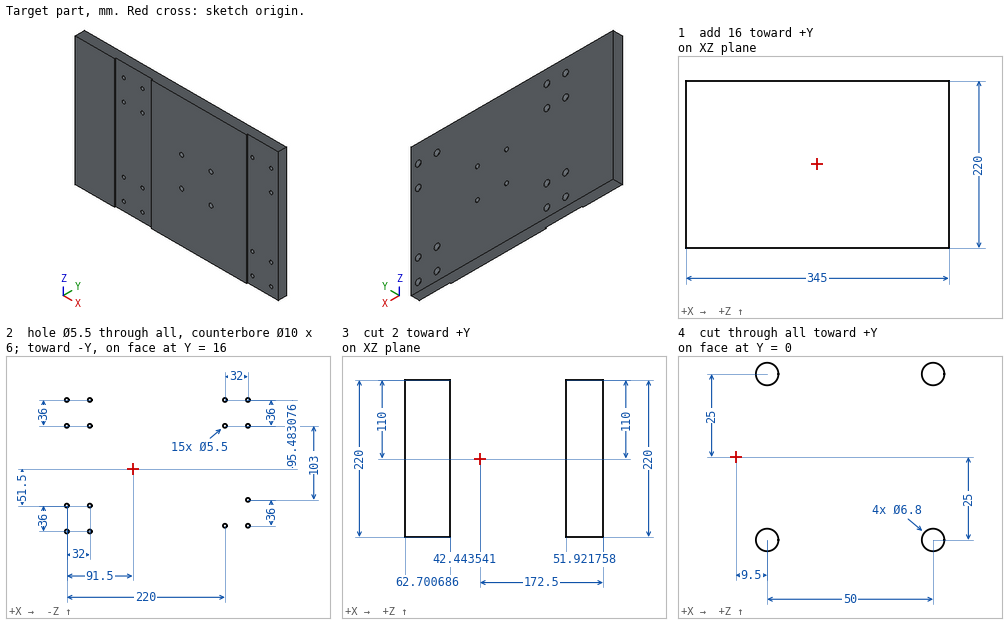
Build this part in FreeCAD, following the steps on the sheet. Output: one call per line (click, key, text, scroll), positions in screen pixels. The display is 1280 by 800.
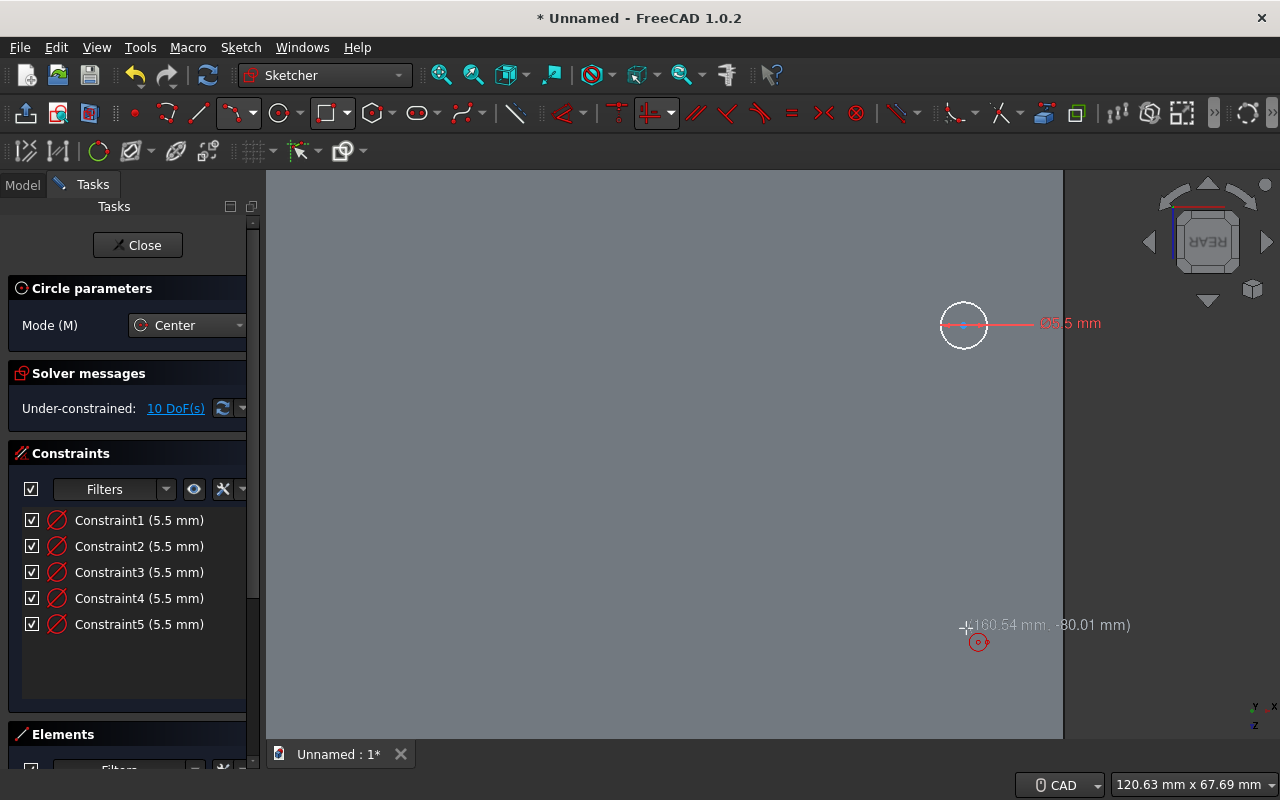
scroll(966, 628, down, 7)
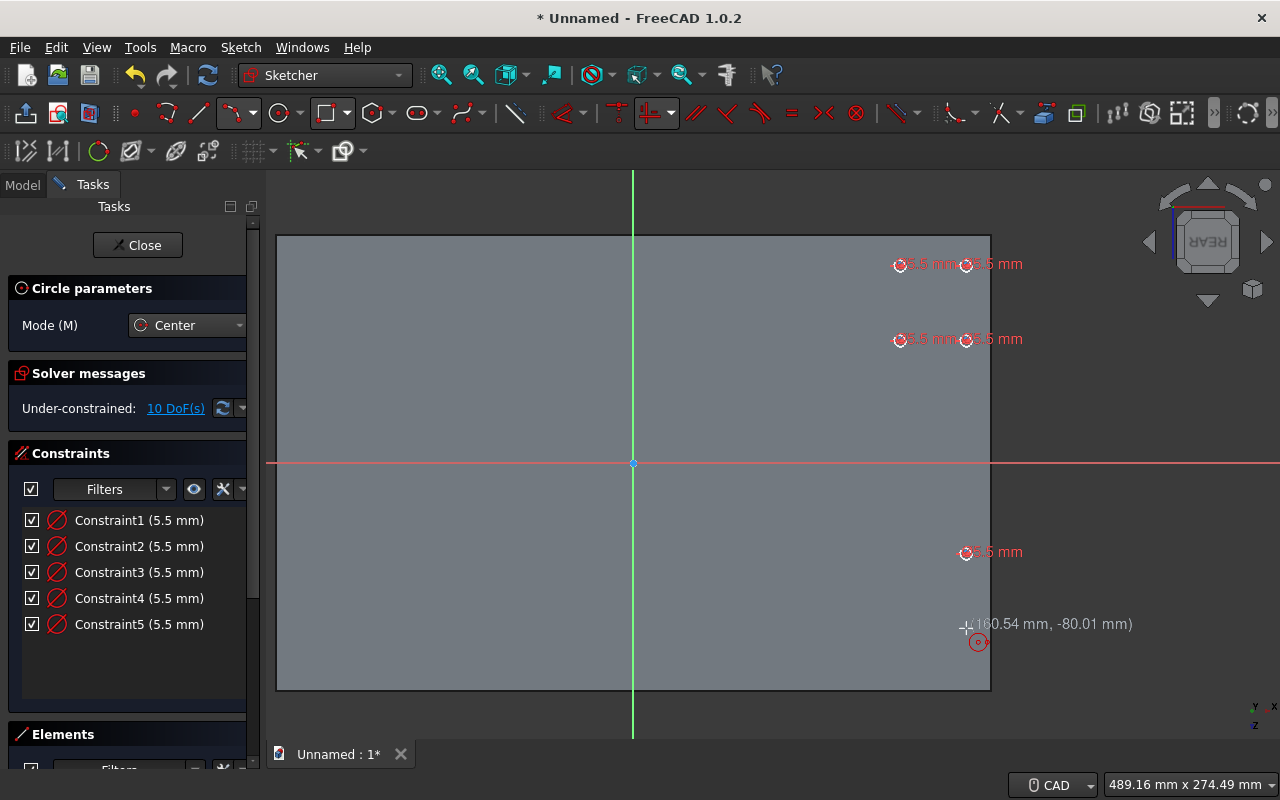
click(966, 628)
move(970, 624)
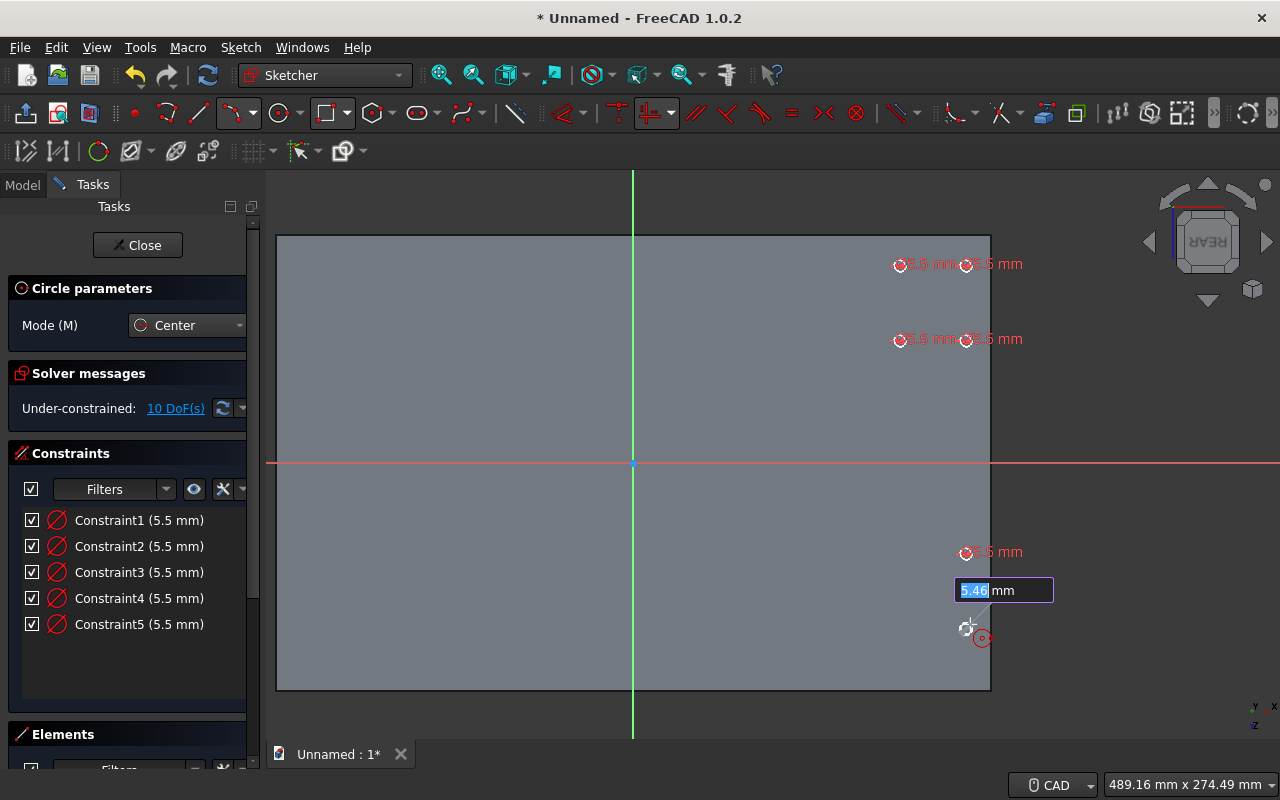
text(5.5)
key(Return)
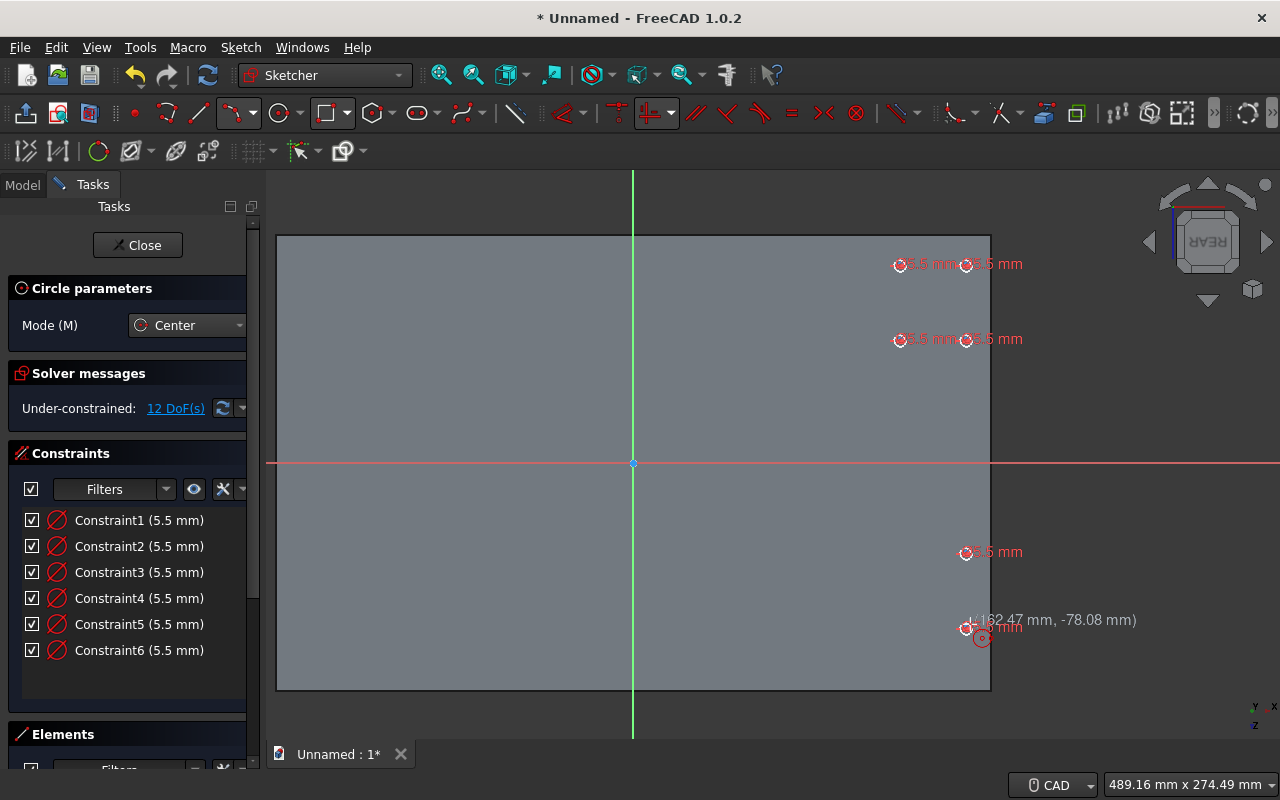
scroll(900, 628, up, 7)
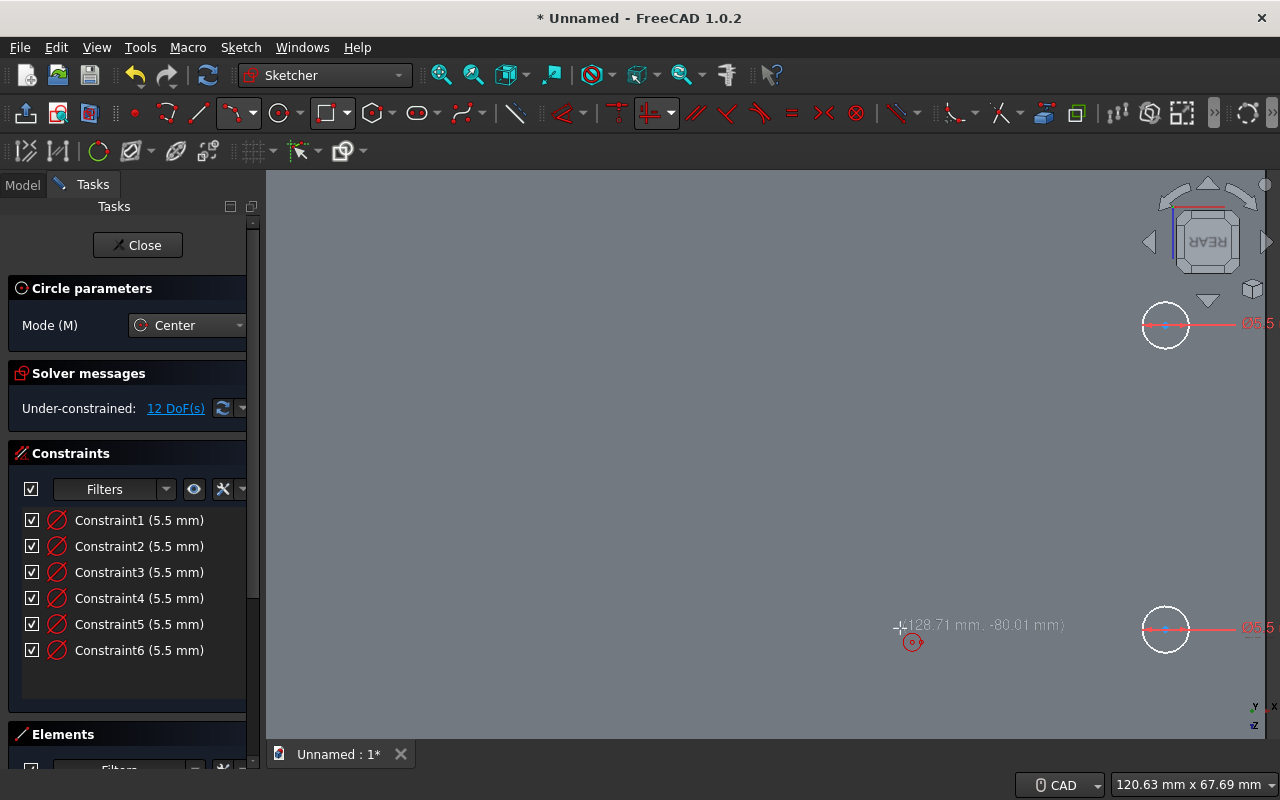
scroll(900, 628, down, 7)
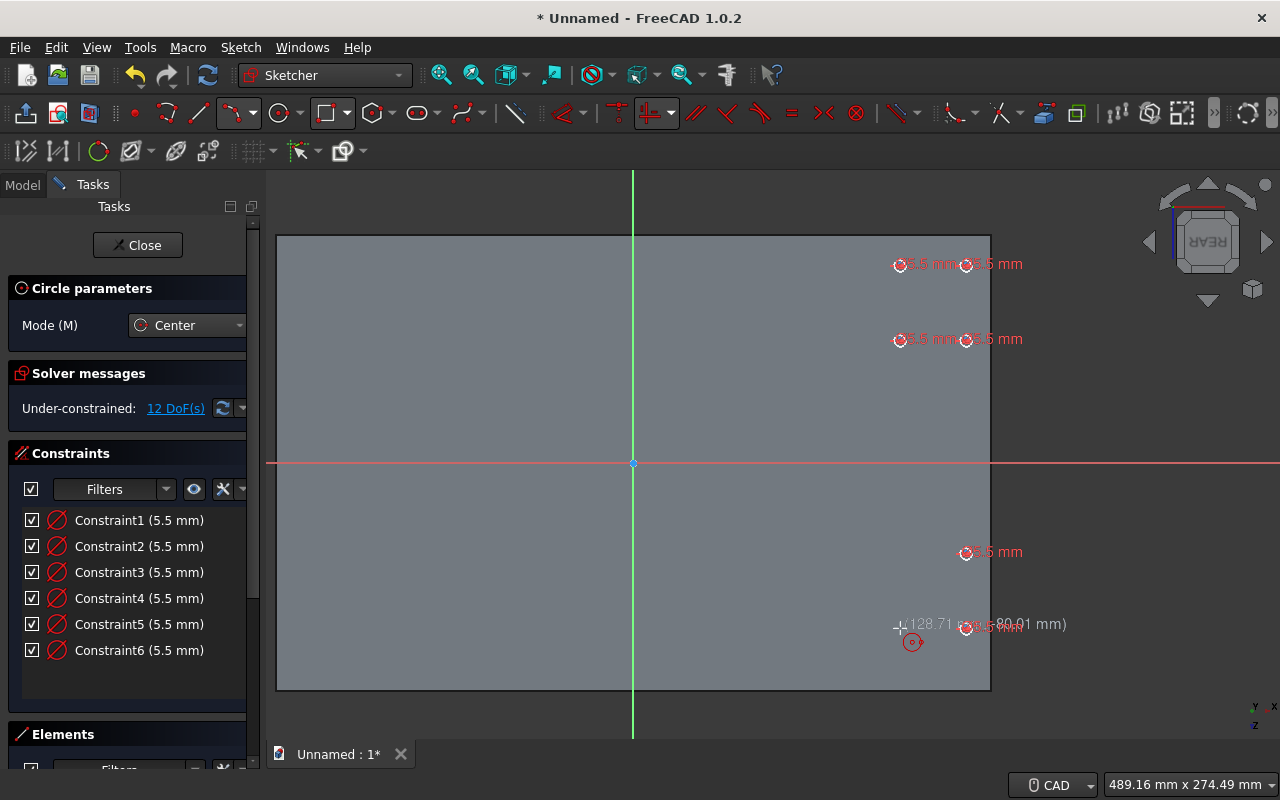
click(900, 628)
move(904, 624)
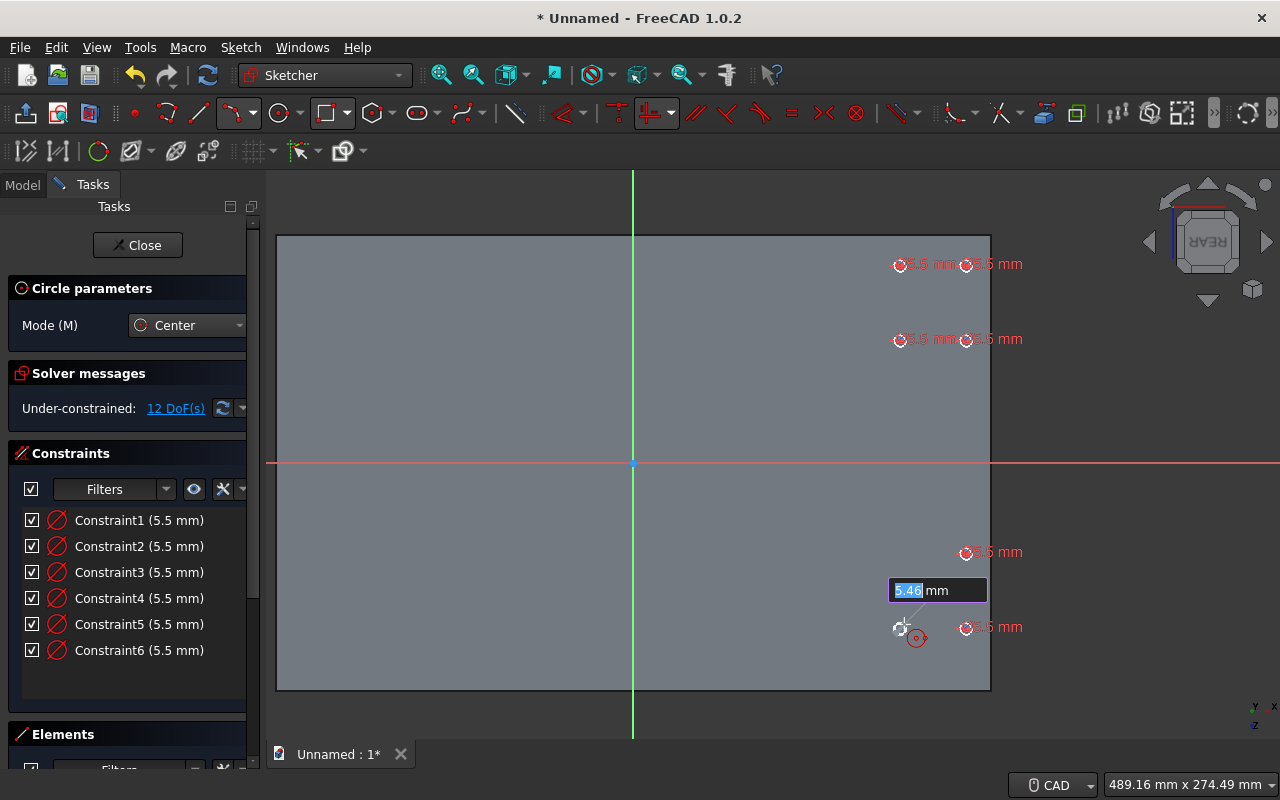
text(5.5)
key(Return)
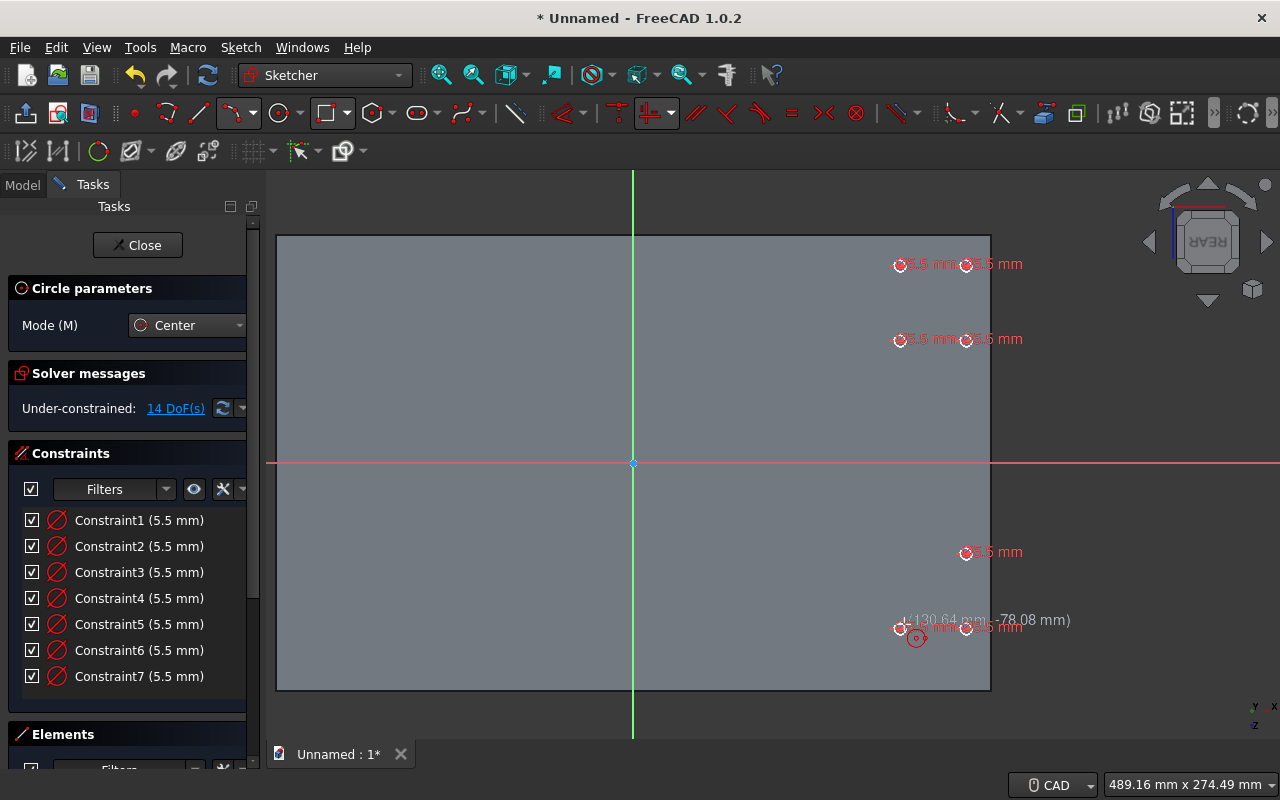
scroll(444, 570, up, 7)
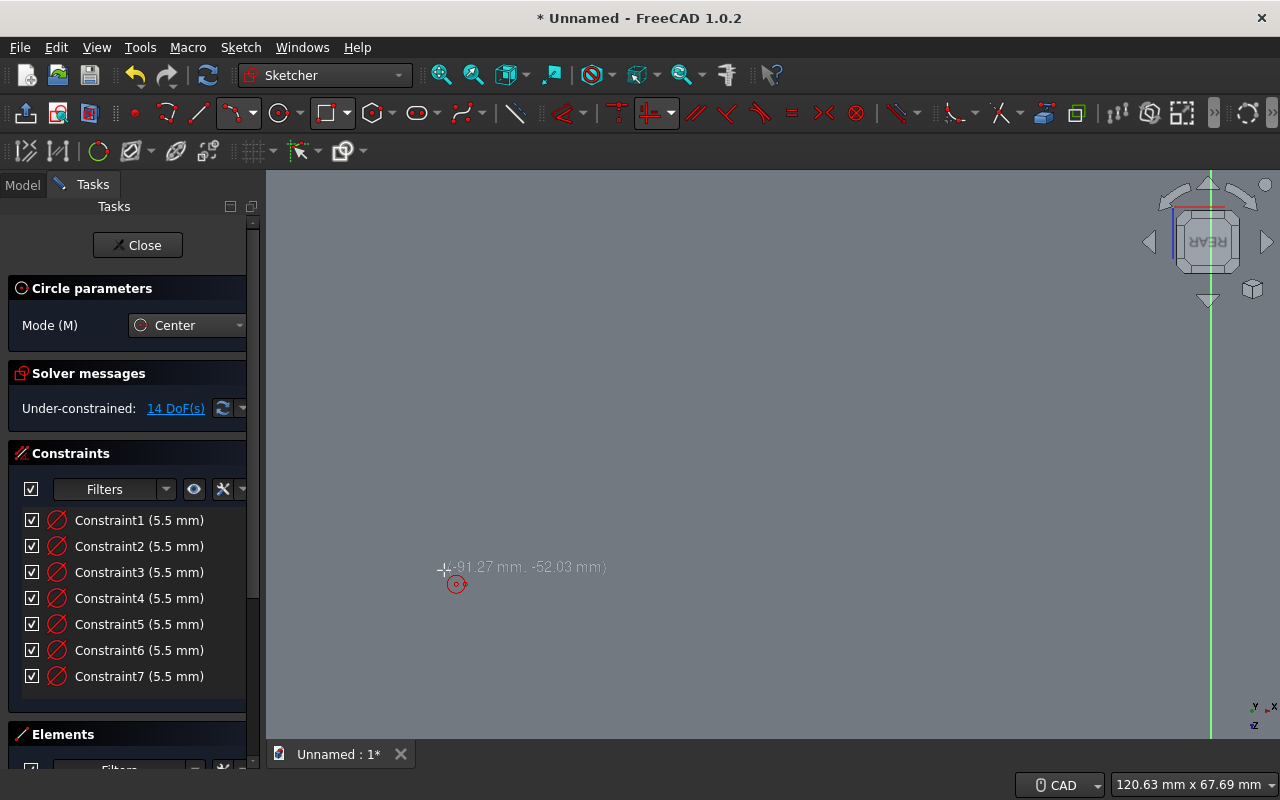
scroll(444, 570, down, 7)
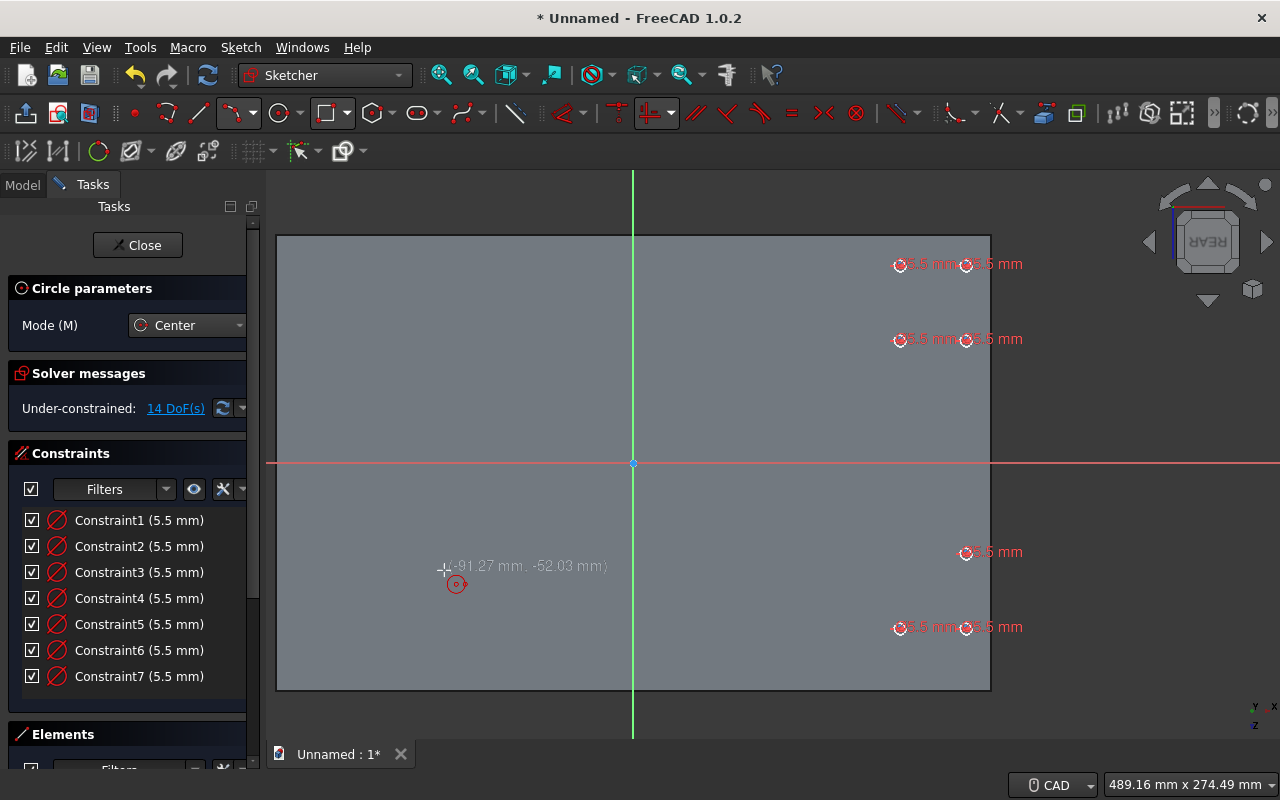
click(444, 570)
move(448, 566)